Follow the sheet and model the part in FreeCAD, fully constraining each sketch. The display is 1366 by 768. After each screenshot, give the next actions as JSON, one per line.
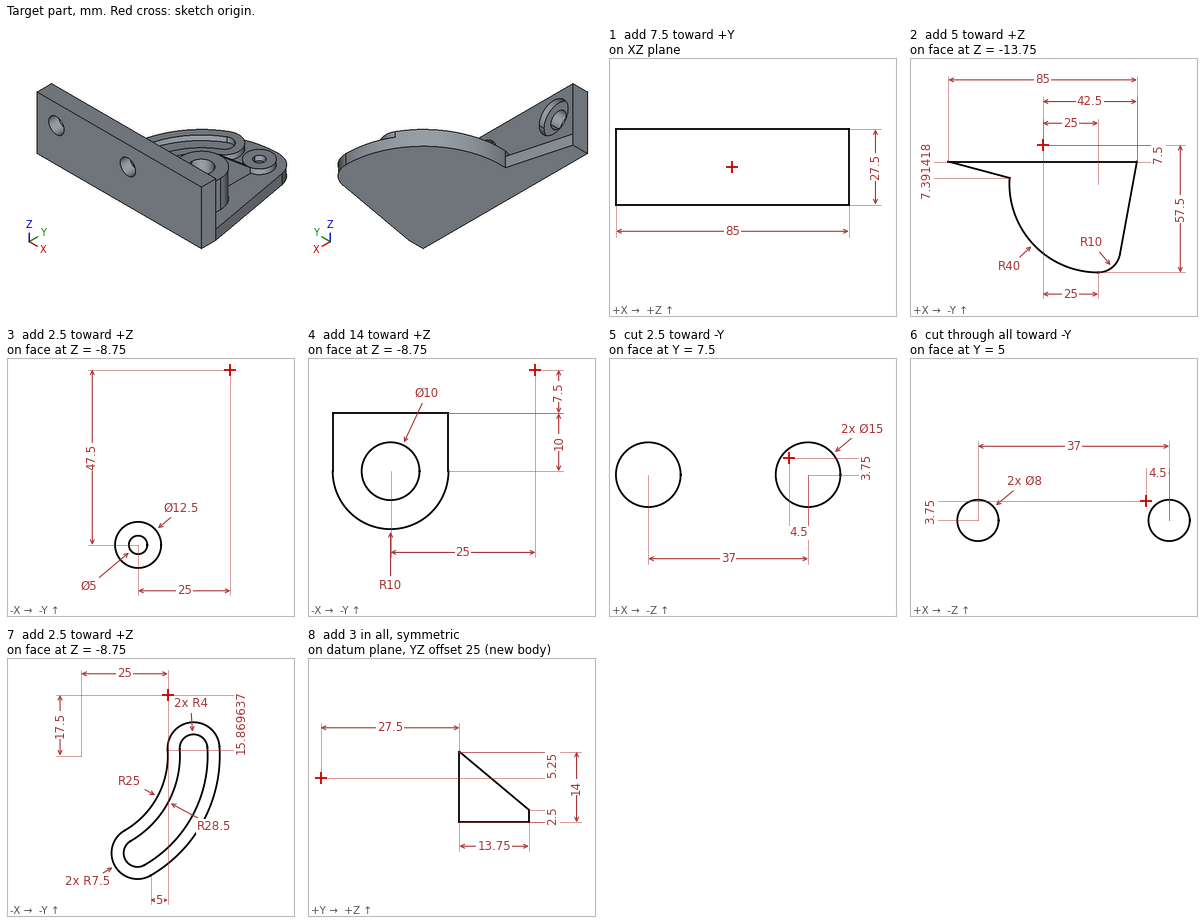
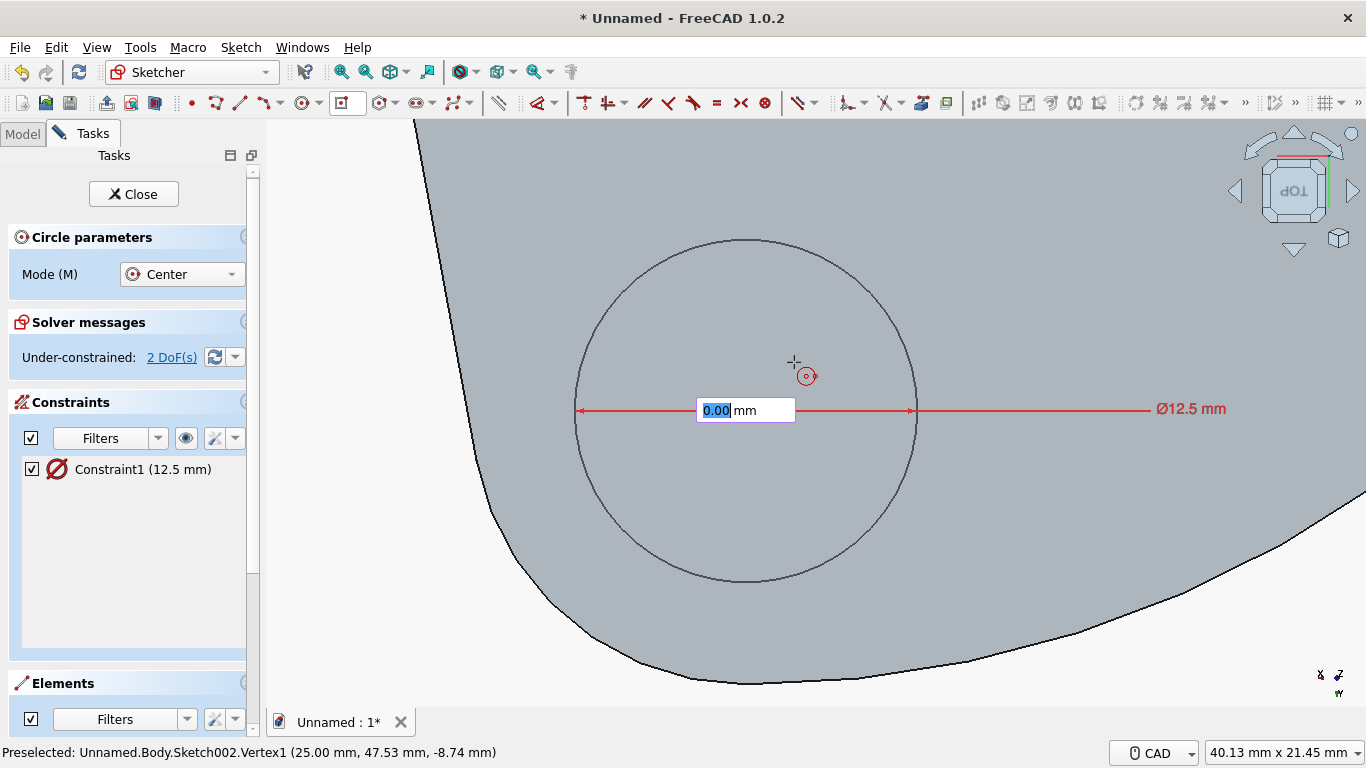
{"action": "type", "text": "5"}
{"action": "key", "text": "Return"}
{"action": "key", "text": "Escape"}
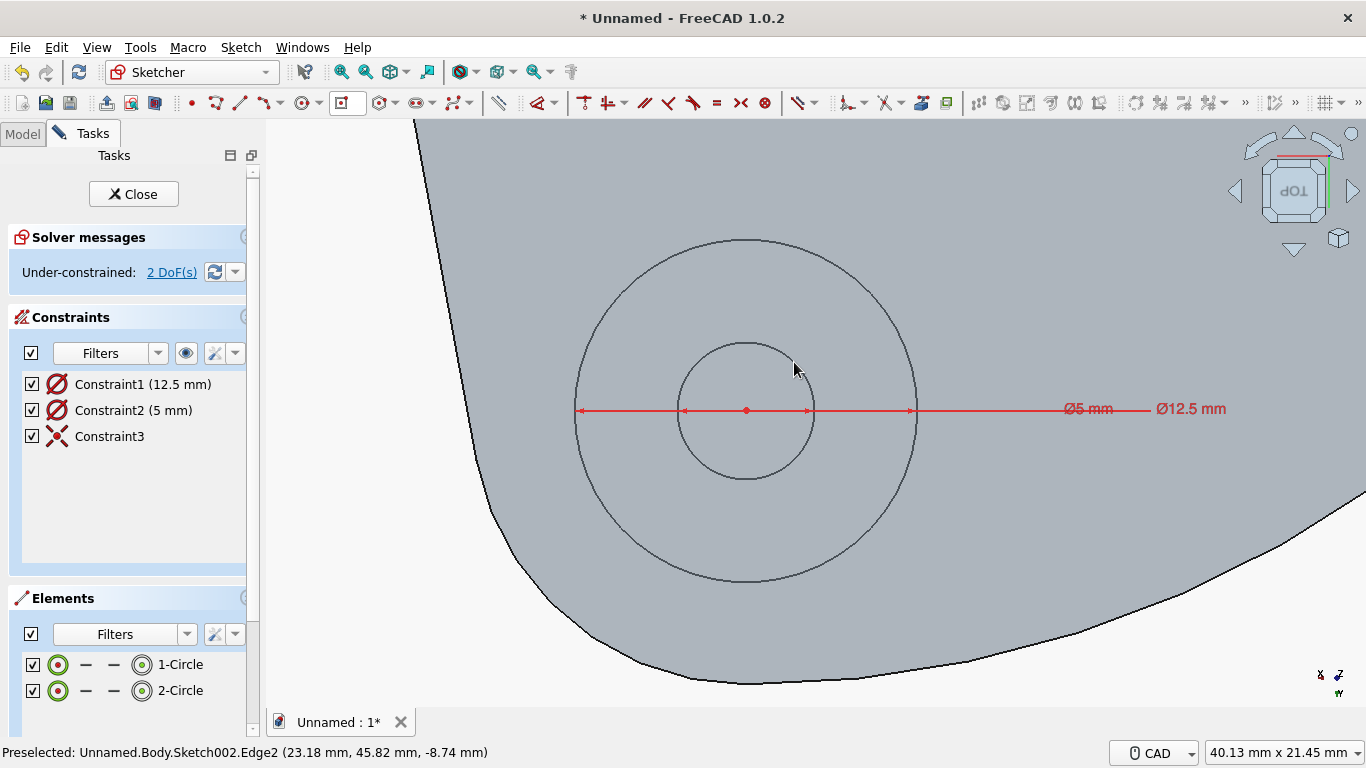
{"action": "left_click", "coordinate": [538, 104]}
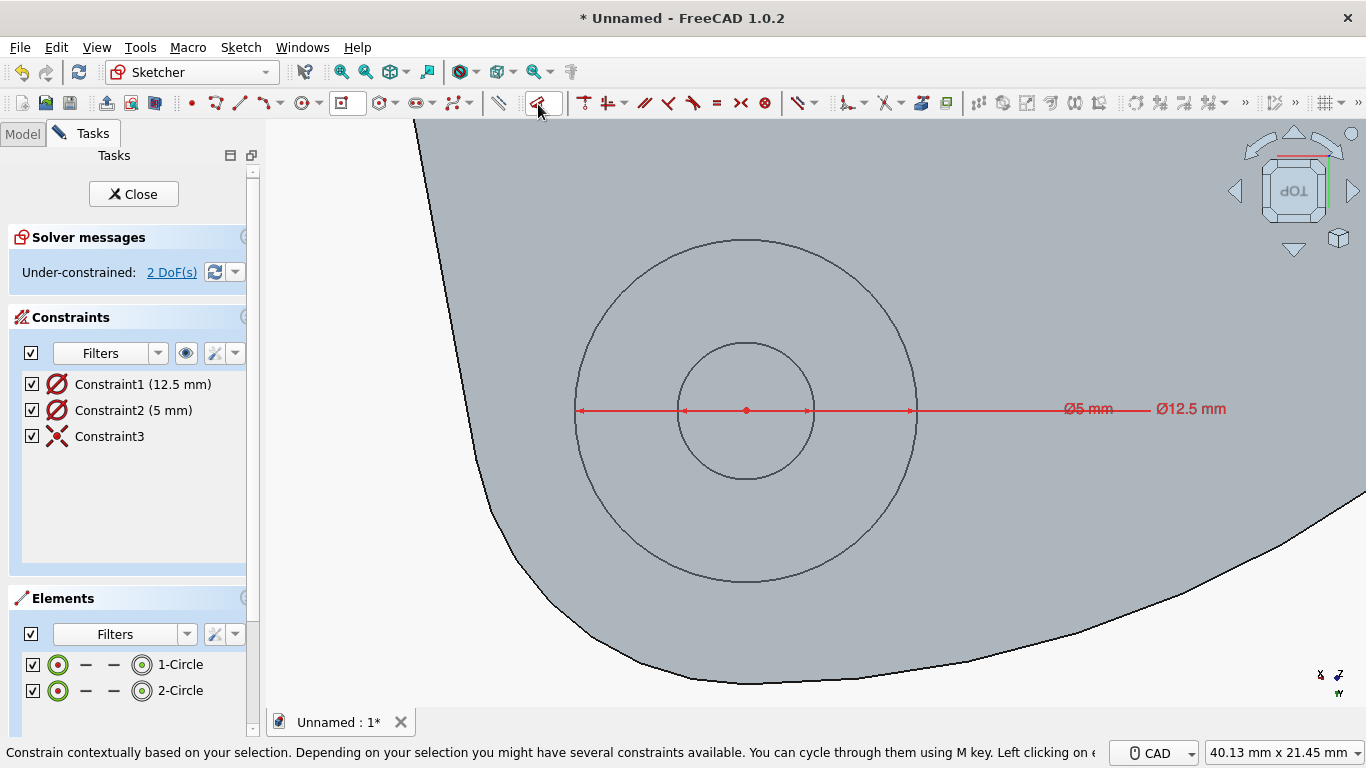
{"action": "left_click", "coordinate": [746, 411]}
{"action": "left_click", "coordinate": [974, 445]}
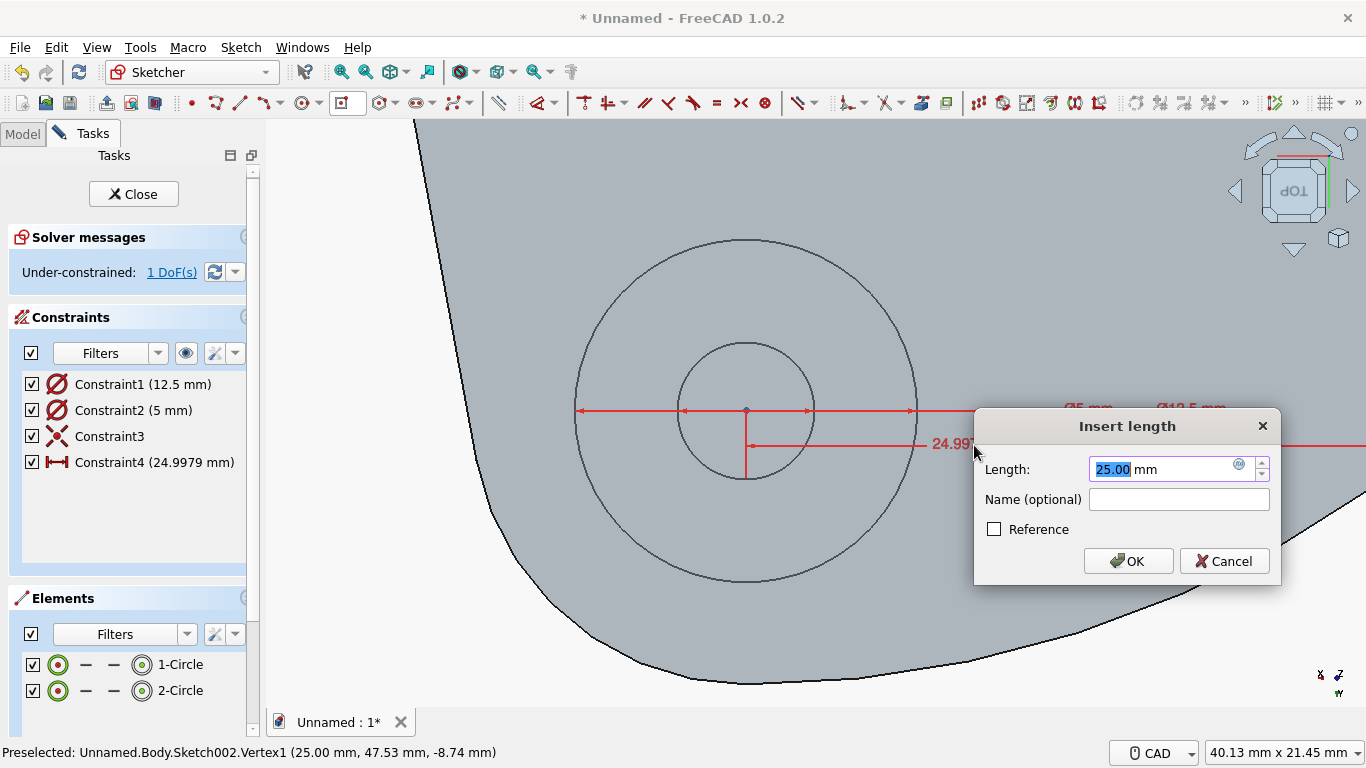
{"action": "type", "text": "25"}
{"action": "key", "text": "Return"}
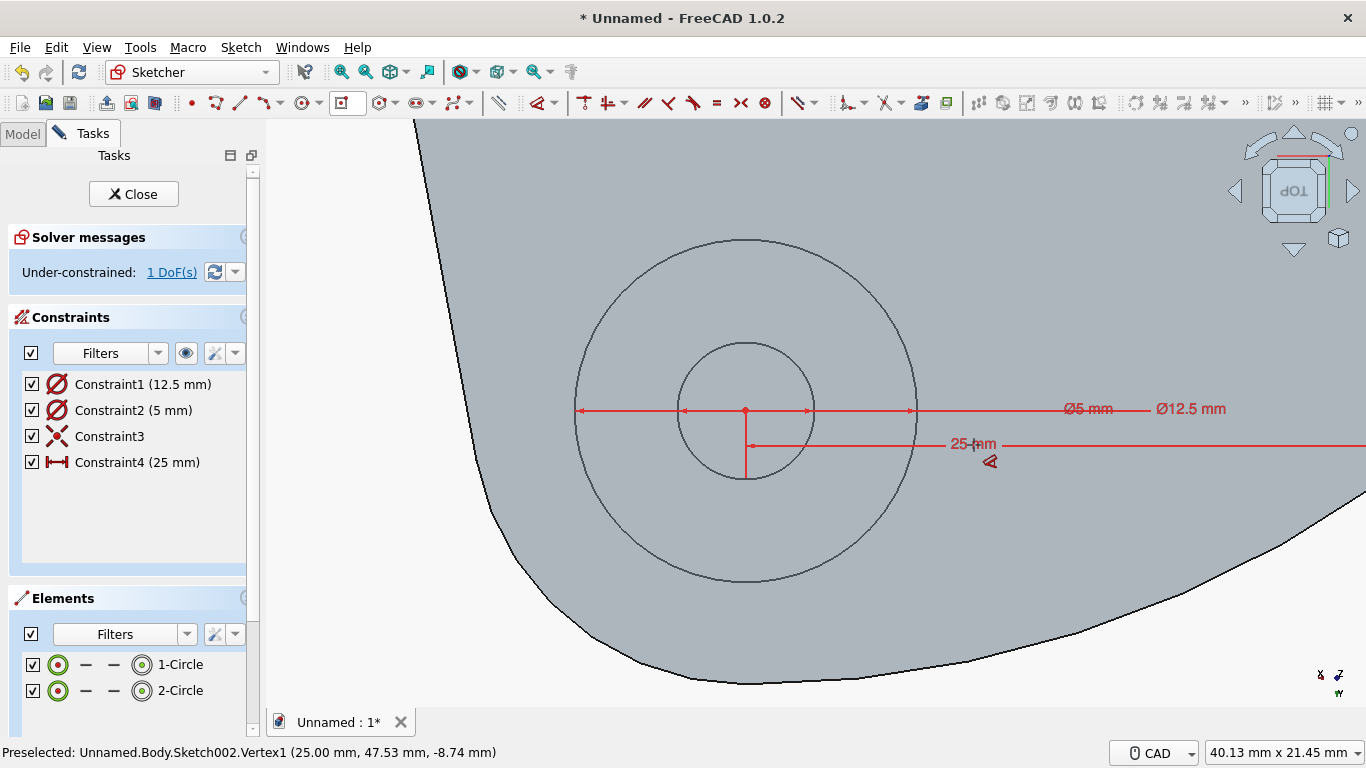
{"action": "left_click", "coordinate": [746, 411]}
{"action": "left_click", "coordinate": [712, 279]}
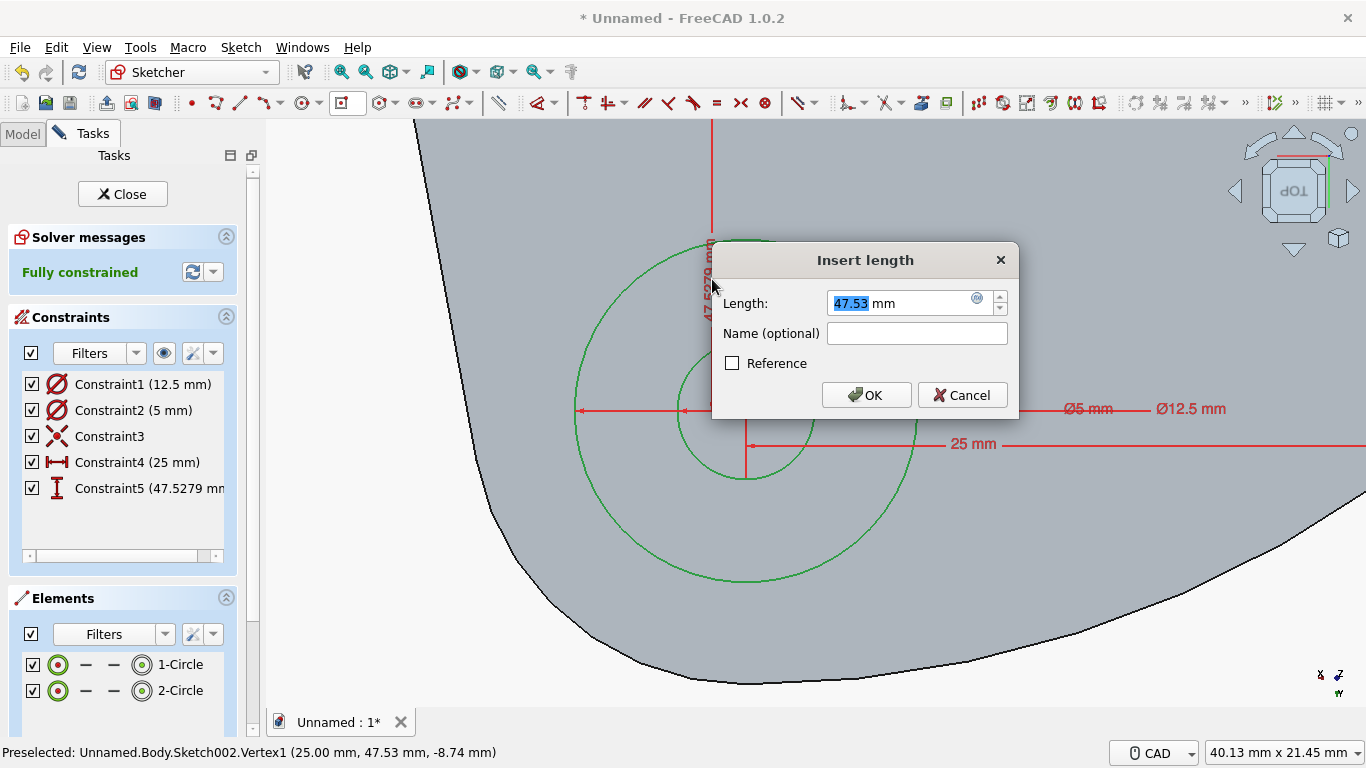
{"action": "type", "text": "47.5"}
{"action": "key", "text": "Return"}
{"action": "key", "text": "Escape"}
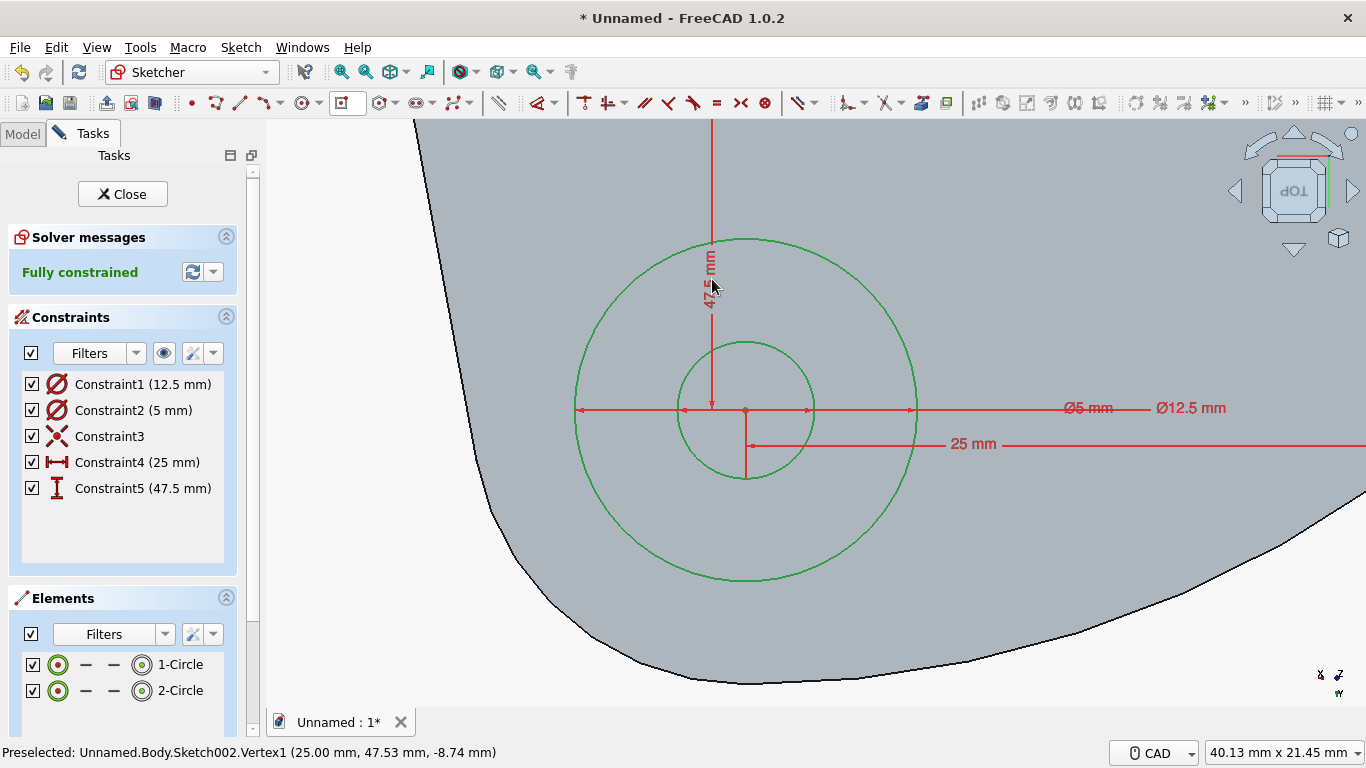
{"action": "left_click", "coordinate": [123, 194]}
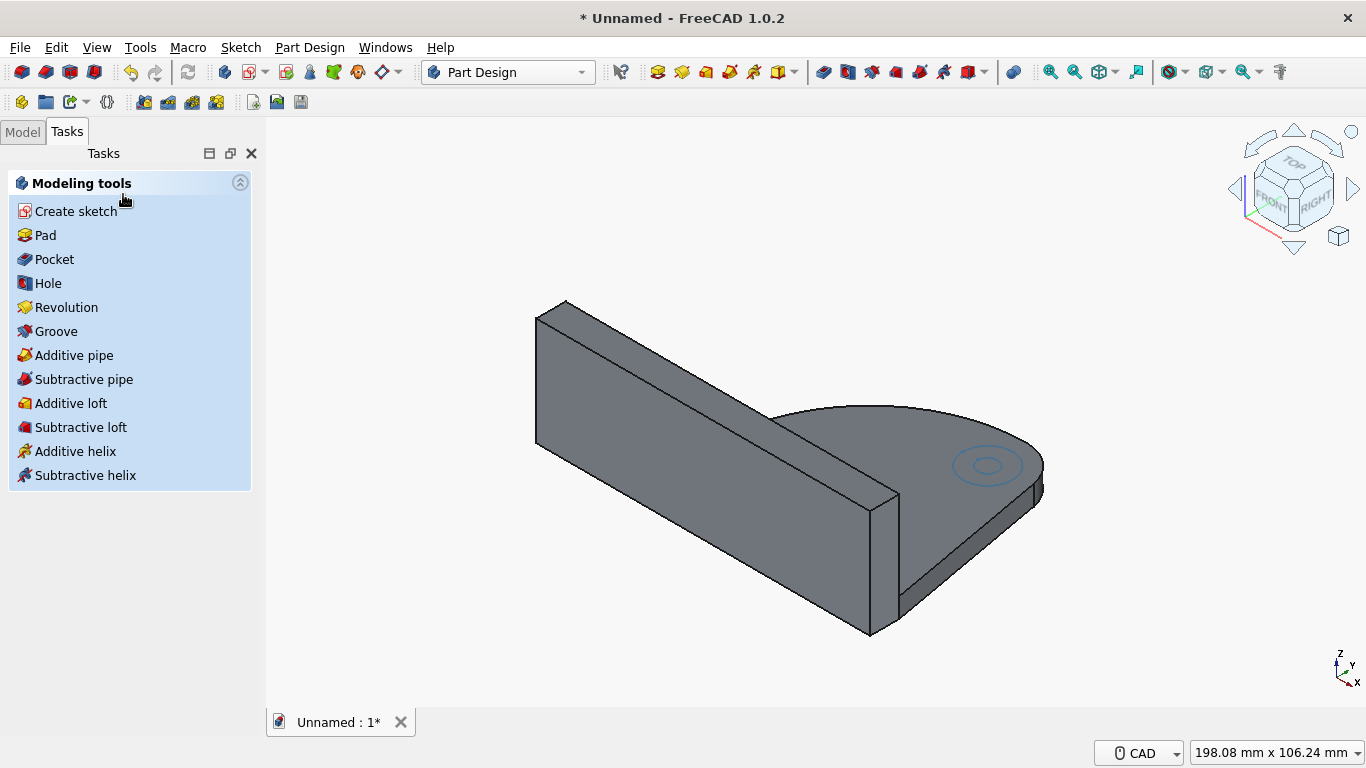
{"action": "left_click", "coordinate": [658, 72]}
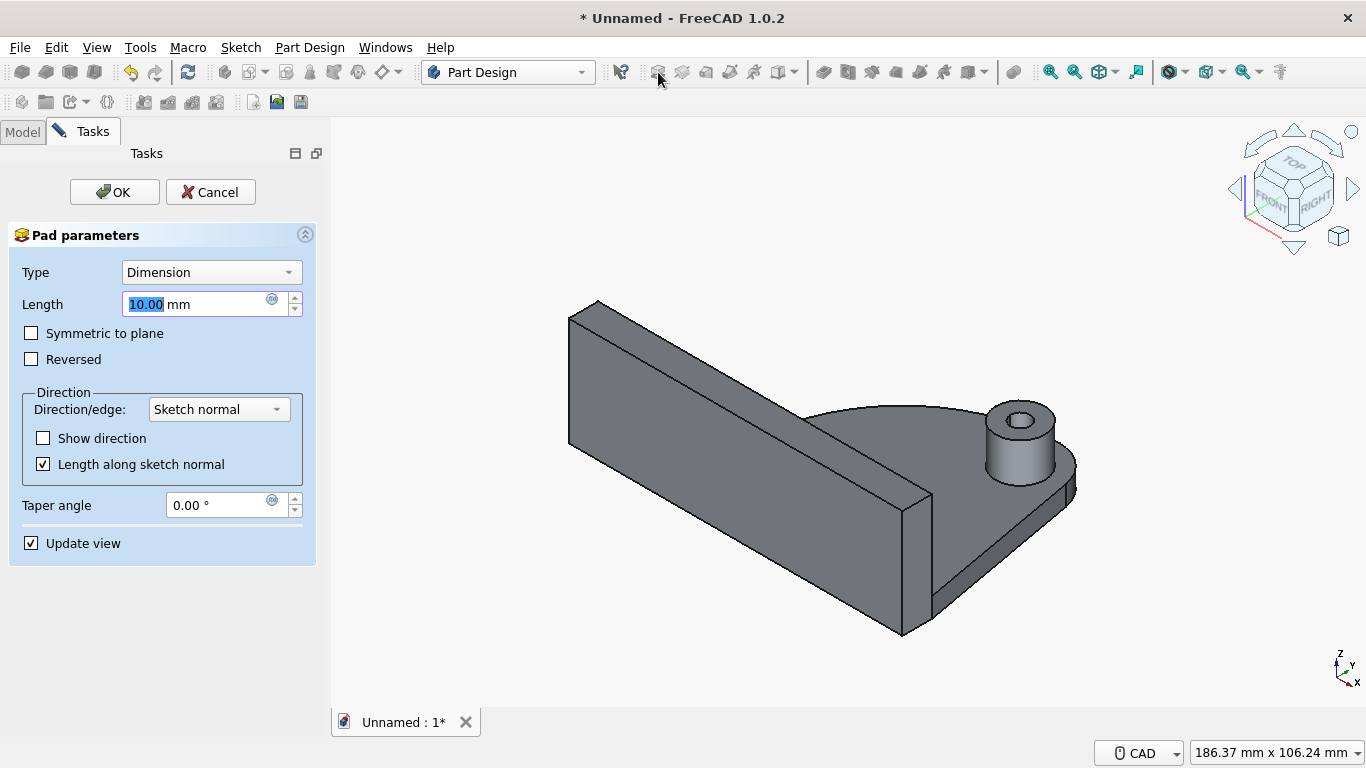
{"action": "type", "text": "2.5"}
{"action": "key", "text": "Tab"}